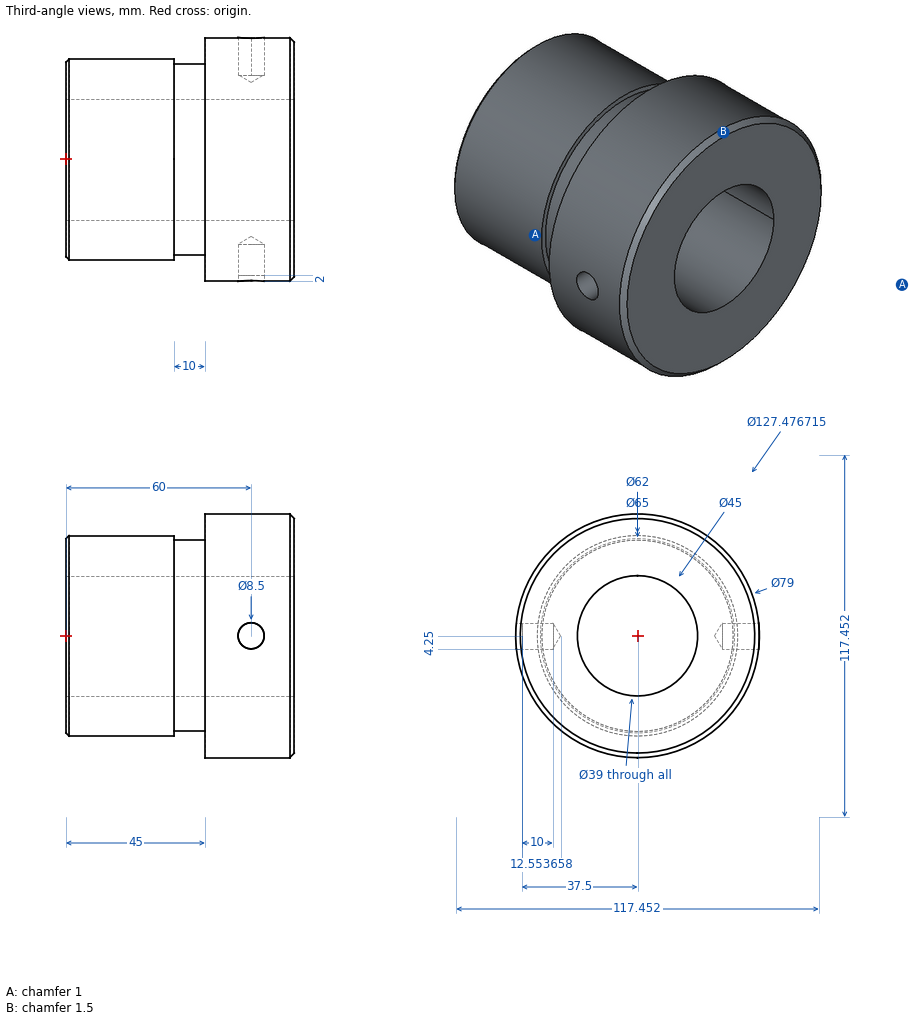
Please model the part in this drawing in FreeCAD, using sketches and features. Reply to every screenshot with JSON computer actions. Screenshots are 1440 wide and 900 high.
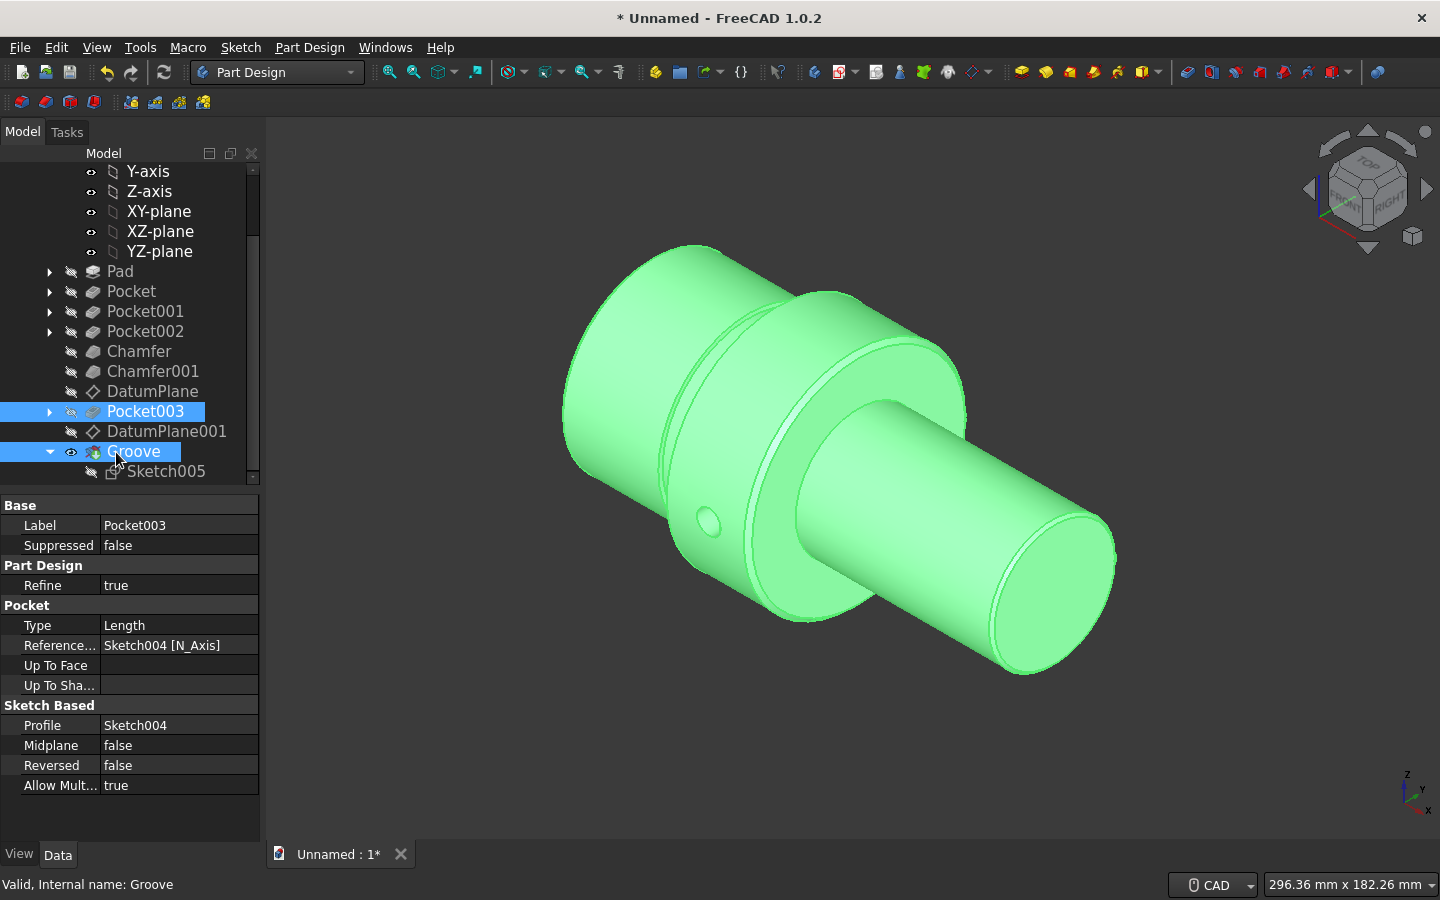
{"action": "left_click", "coordinate": [132, 102]}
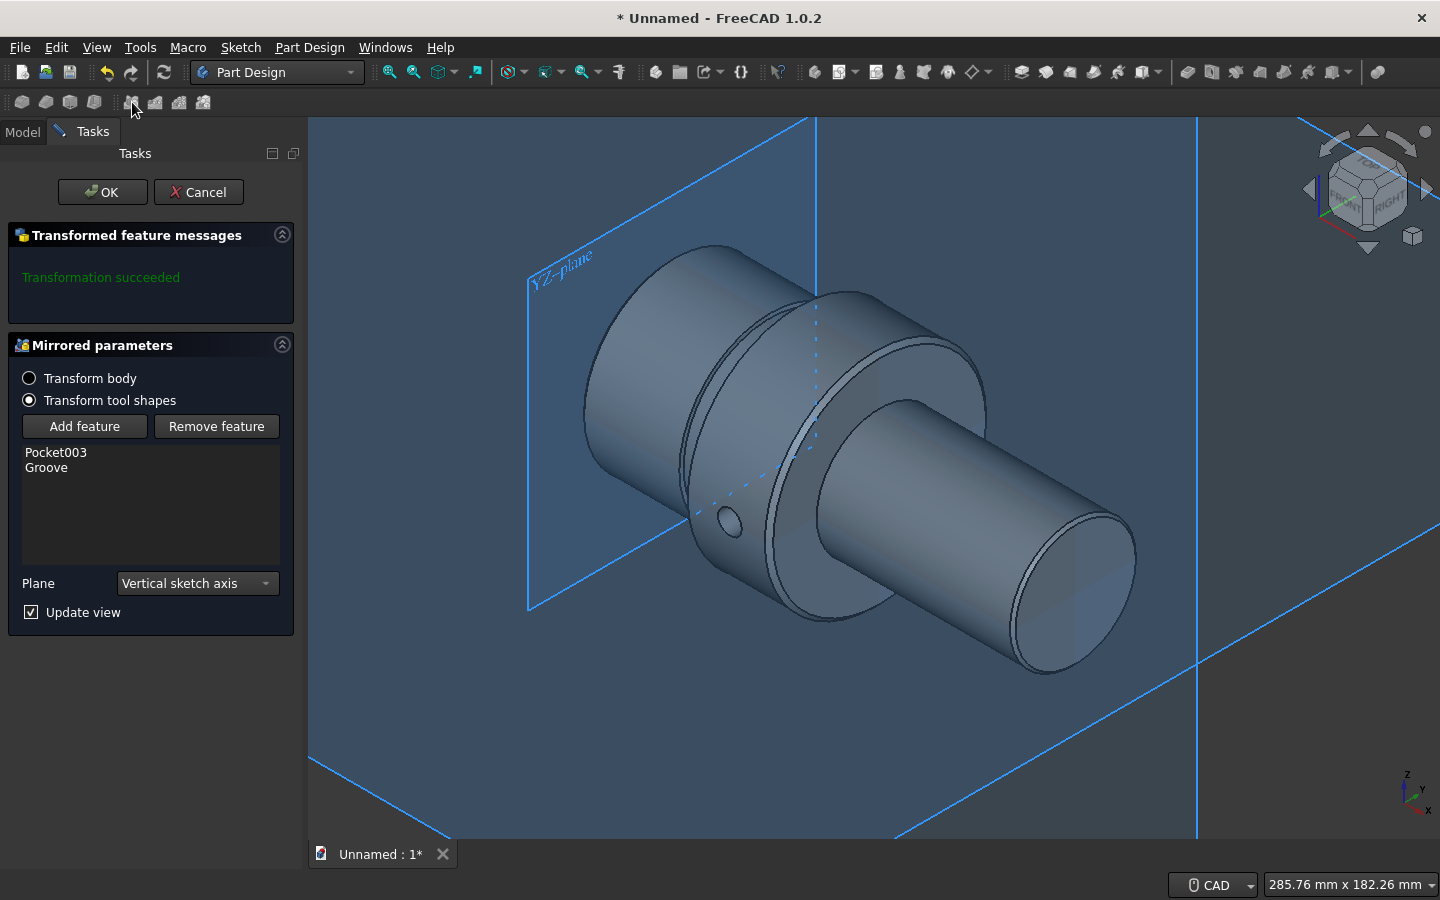
{"action": "left_click", "coordinate": [198, 584]}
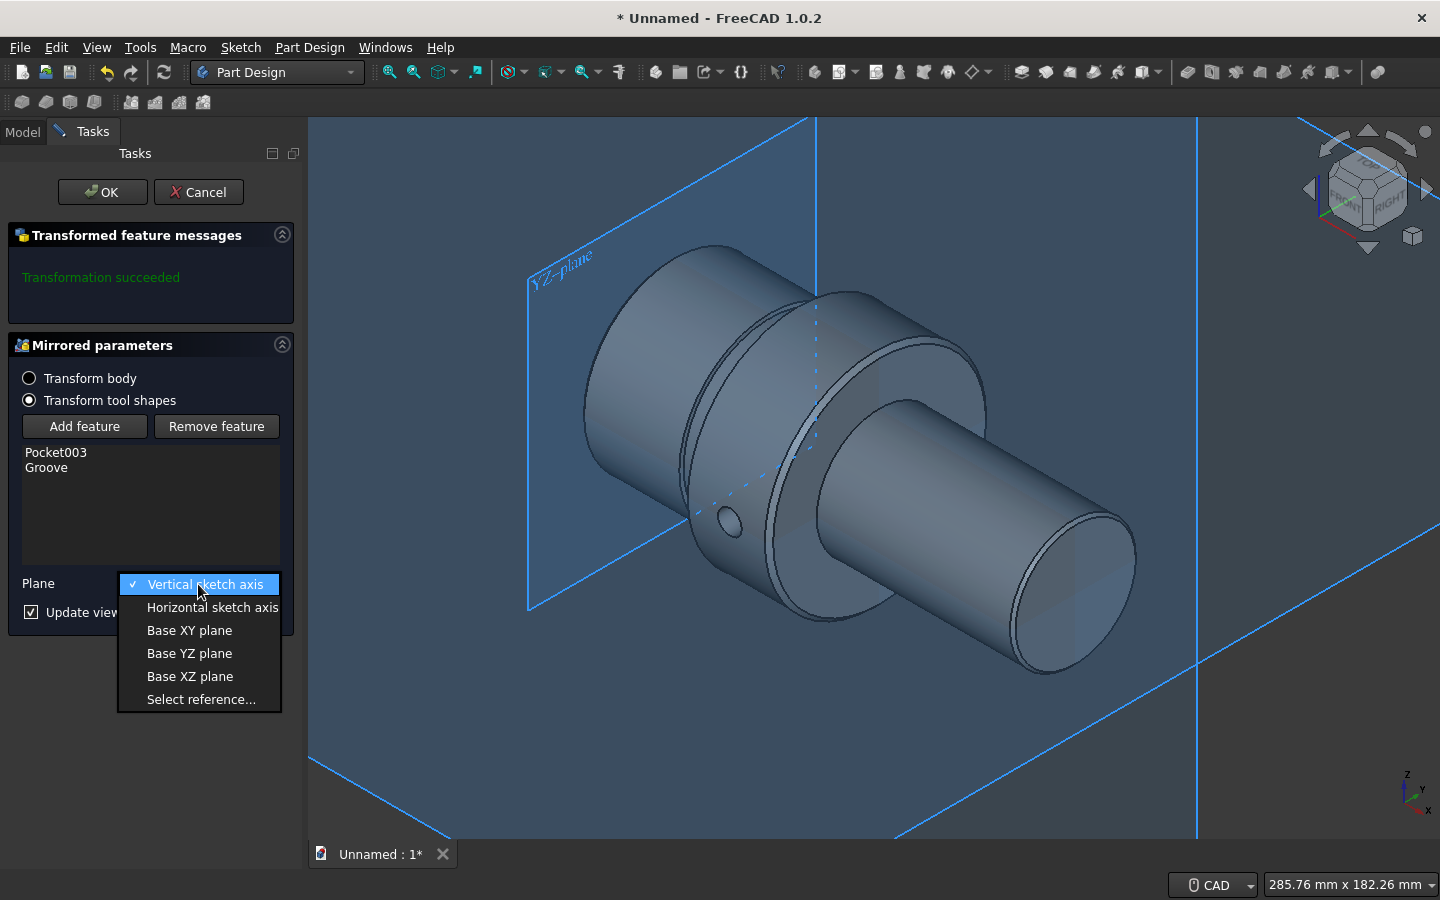
{"action": "left_click", "coordinate": [198, 676]}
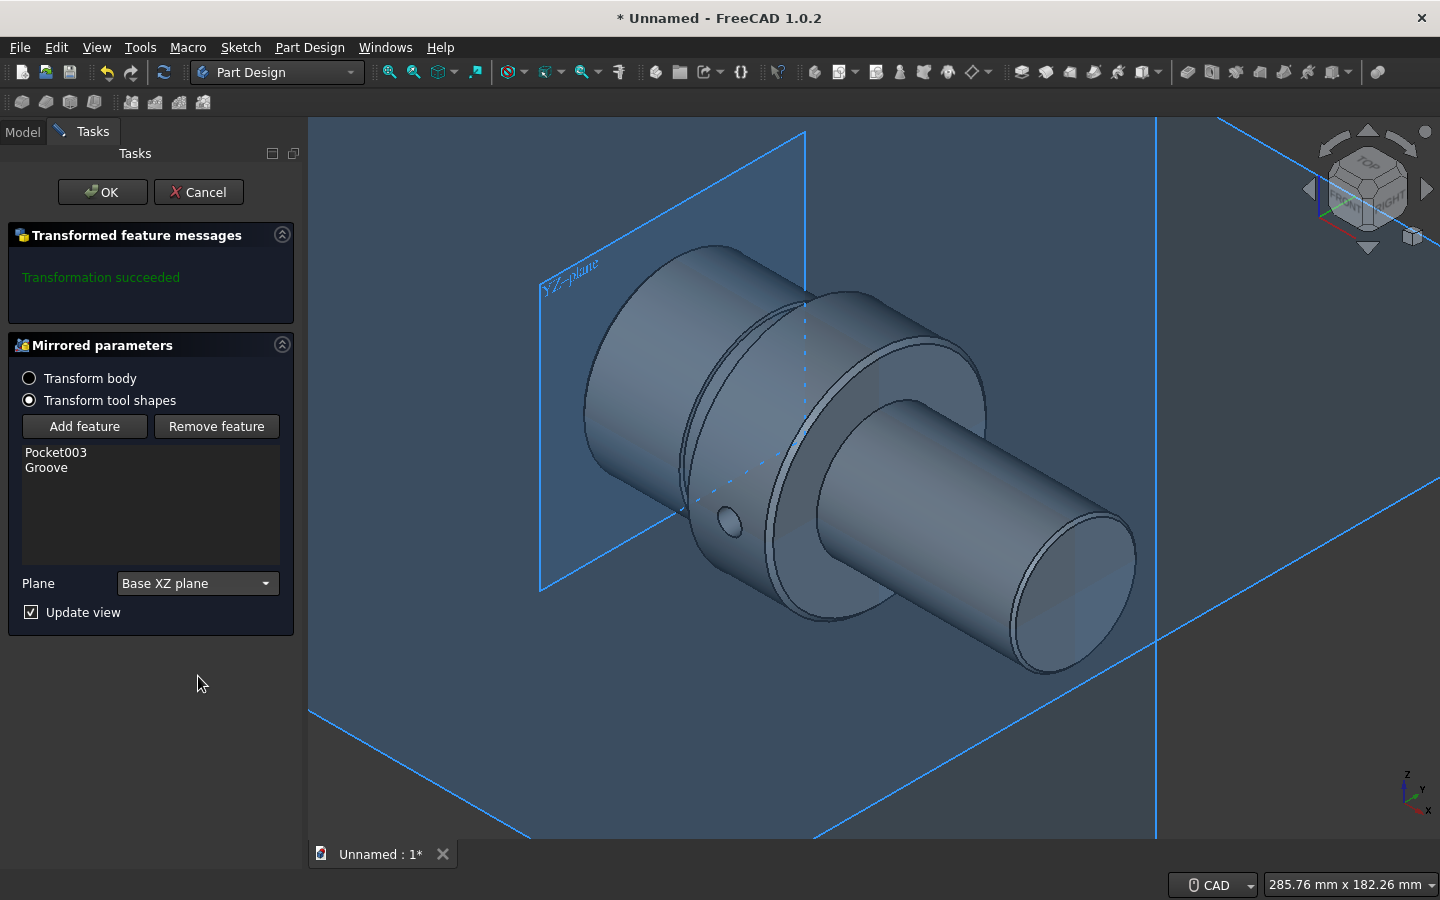
{"action": "left_click", "coordinate": [103, 192]}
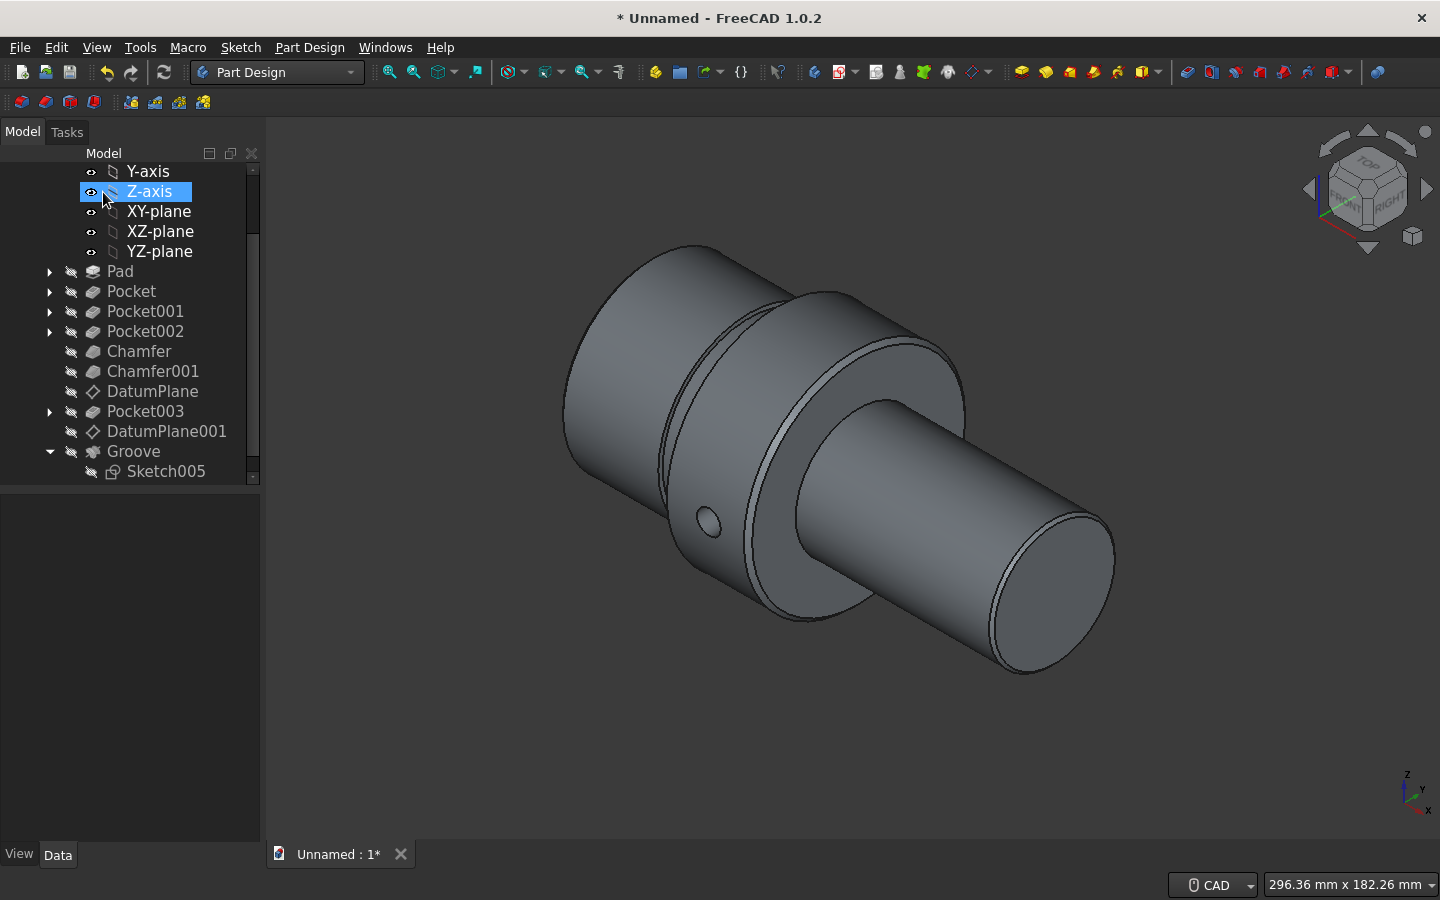
{"action": "left_click", "coordinate": [1055, 593]}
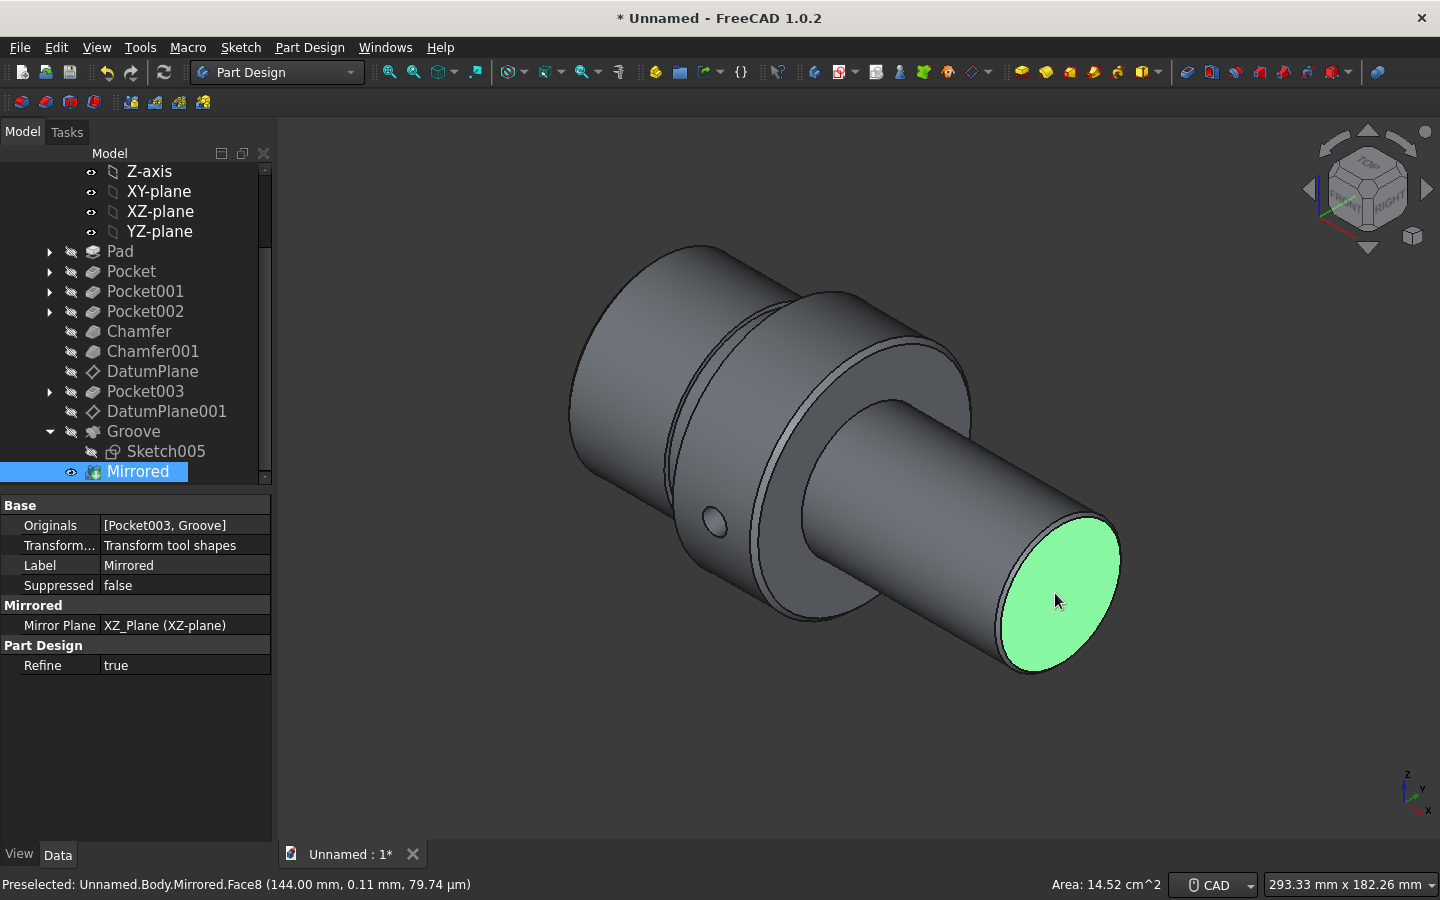
{"action": "left_click", "coordinate": [840, 72]}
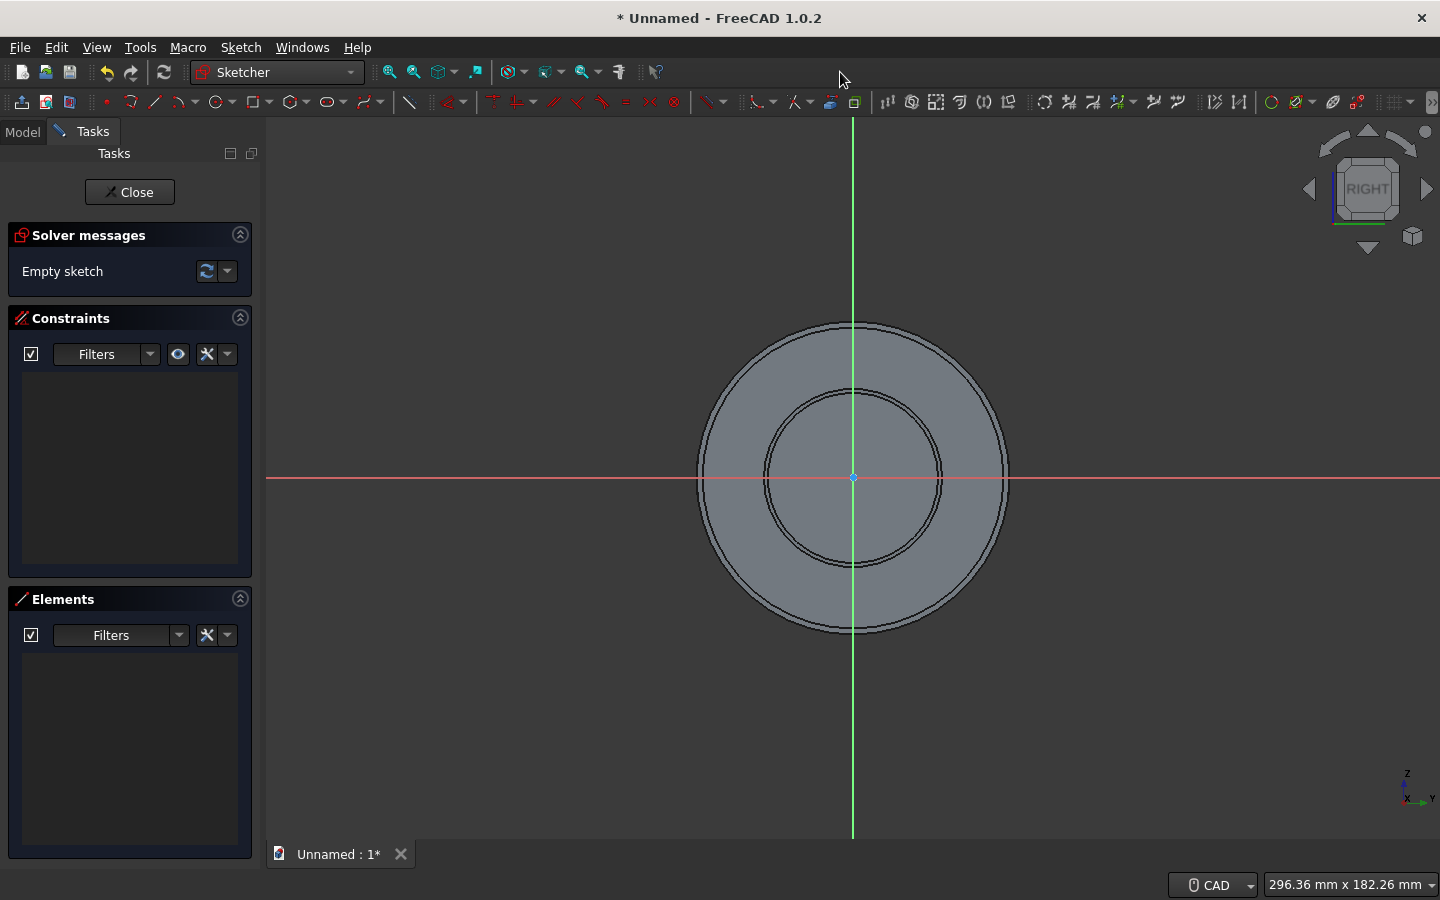
{"action": "key", "text": "g c"}